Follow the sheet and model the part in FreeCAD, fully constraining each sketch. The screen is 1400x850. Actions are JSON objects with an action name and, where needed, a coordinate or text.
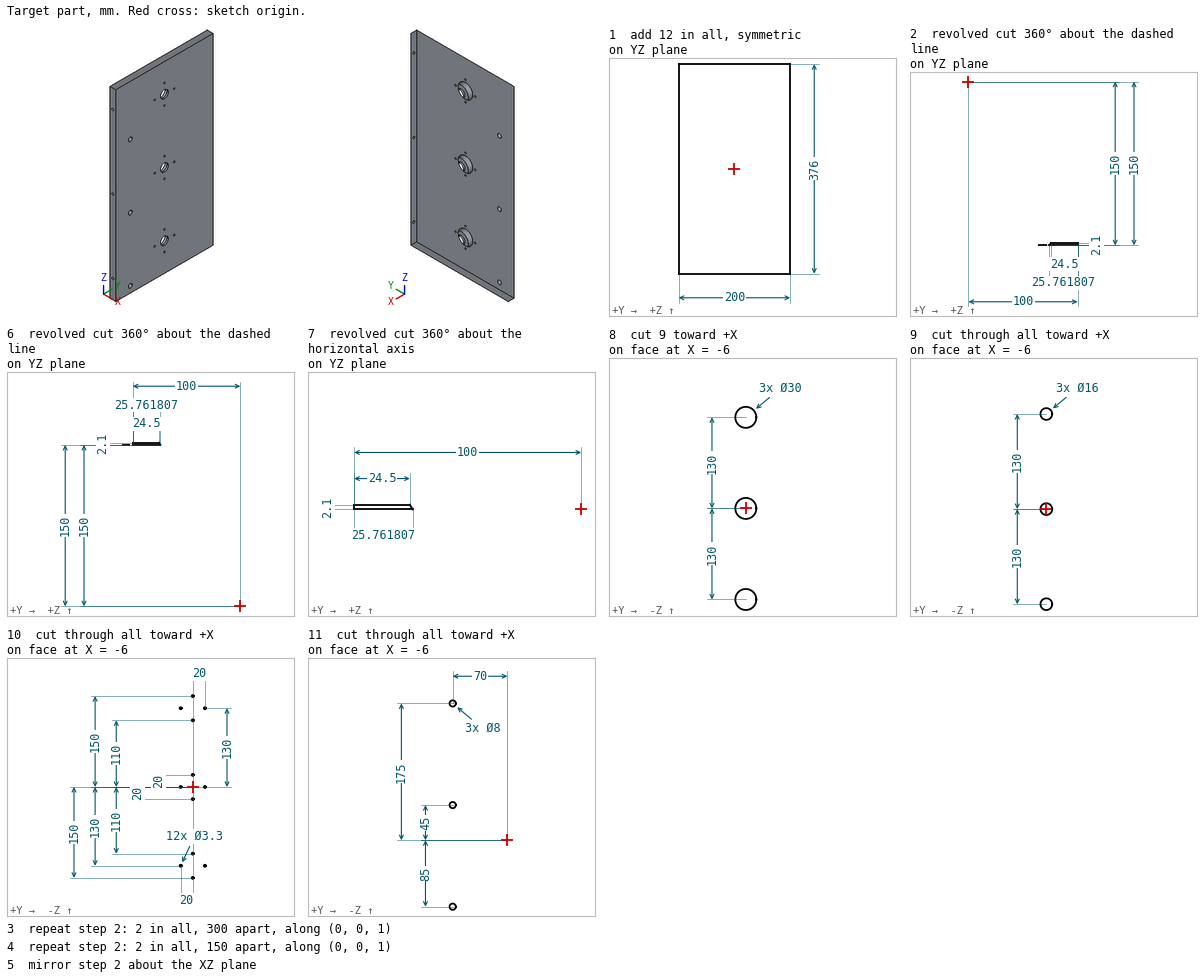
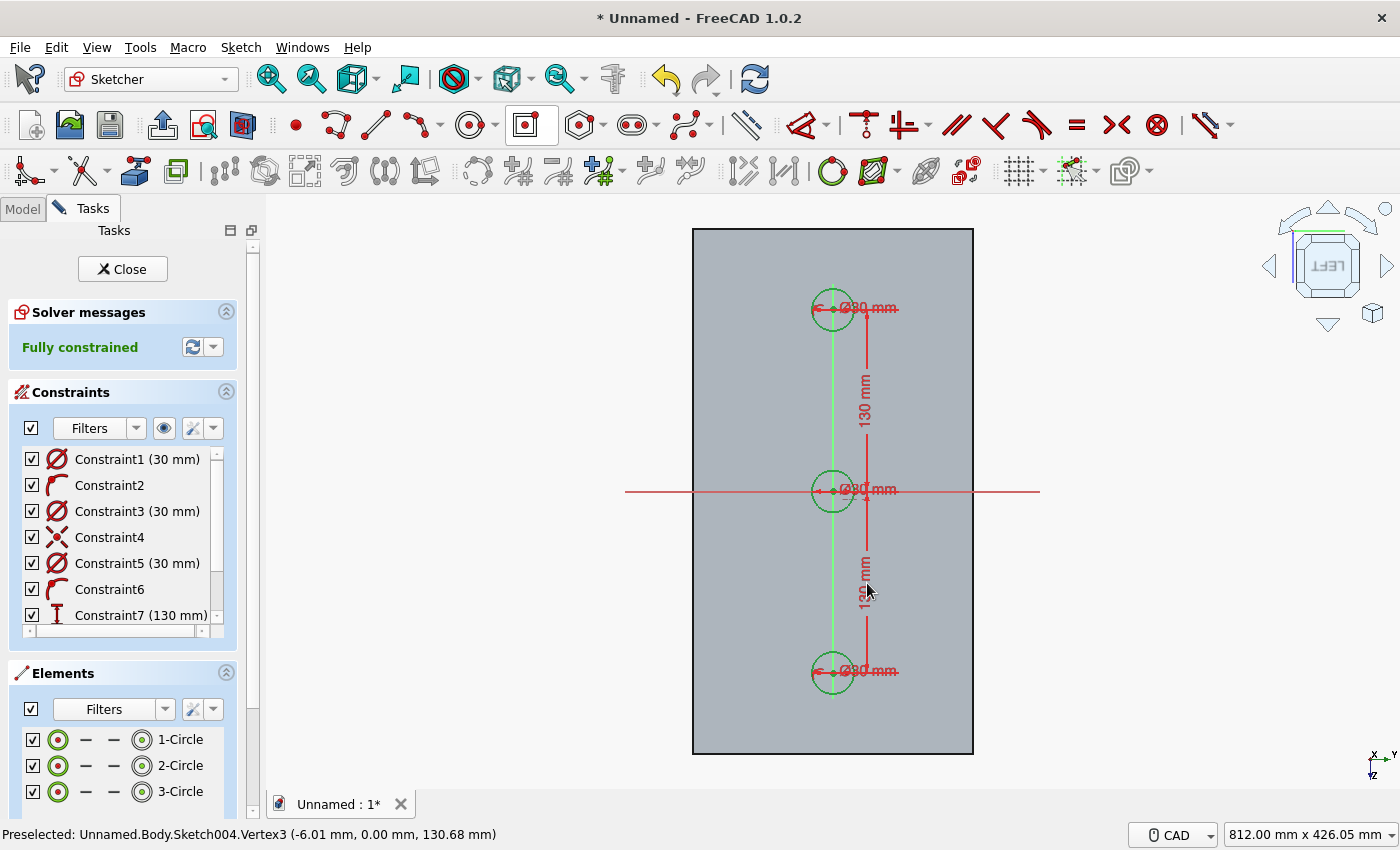
{"action": "left_click", "coordinate": [123, 269]}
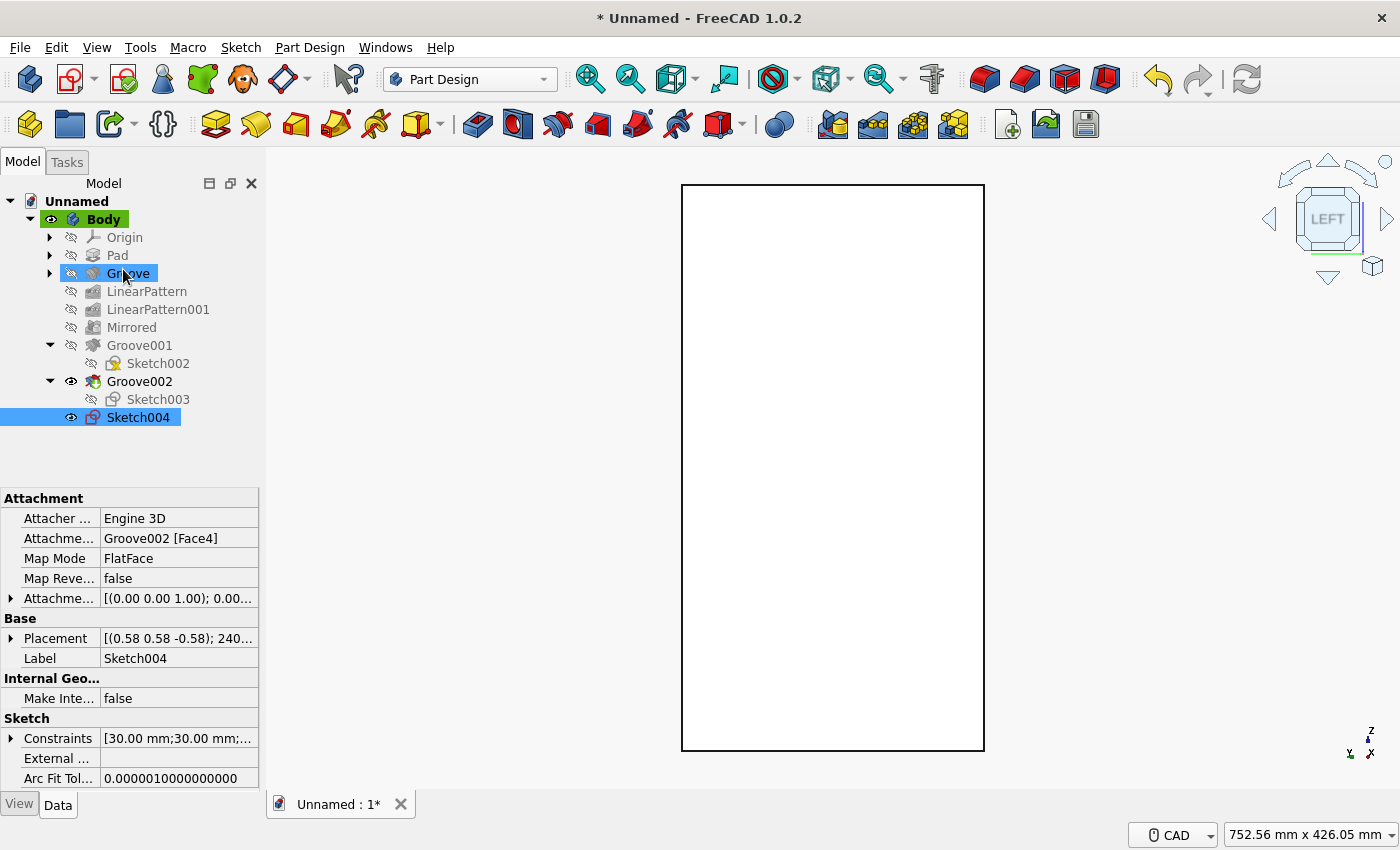
{"action": "left_click", "coordinate": [478, 124]}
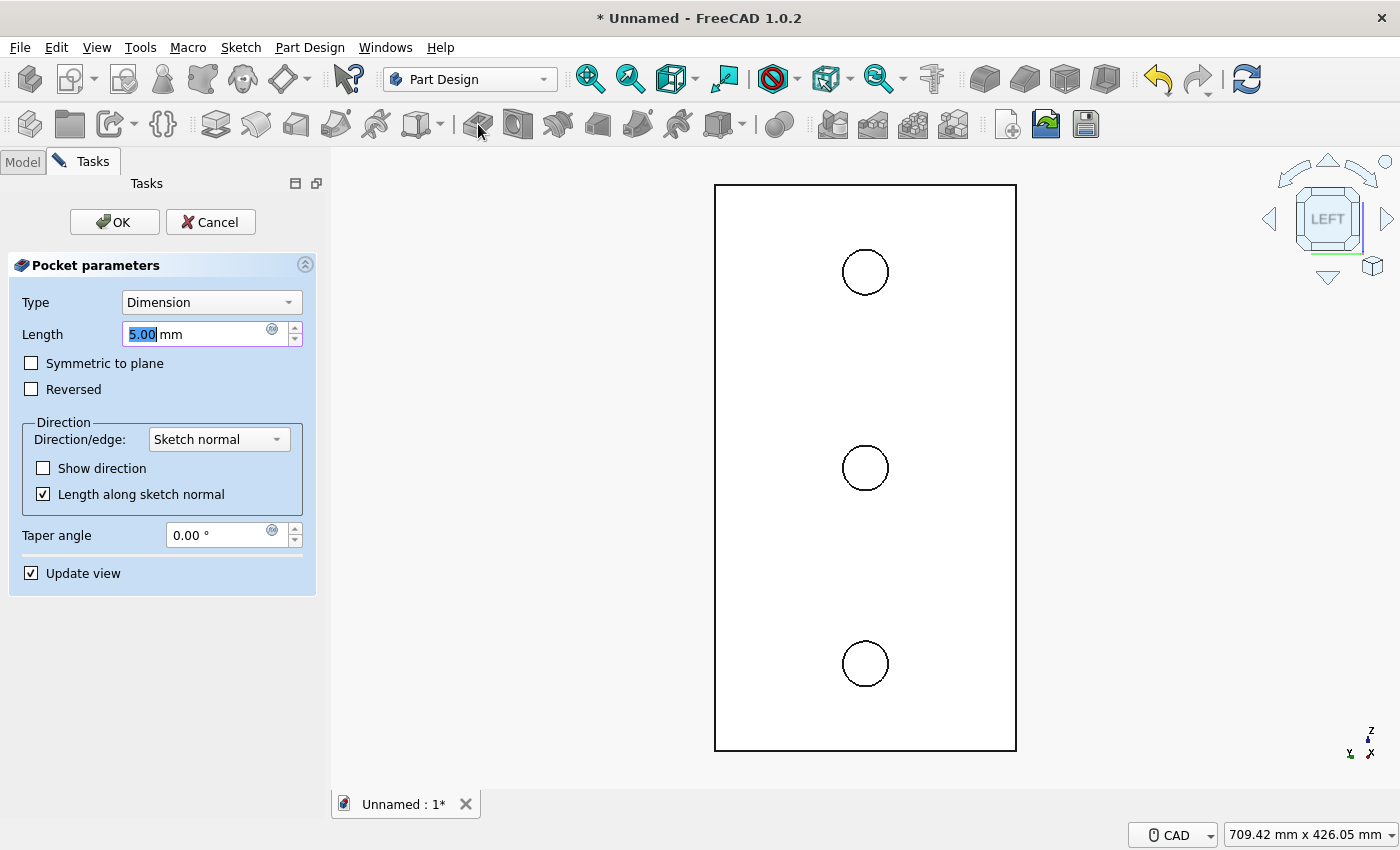
{"action": "type", "text": "9"}
{"action": "key", "text": "Tab"}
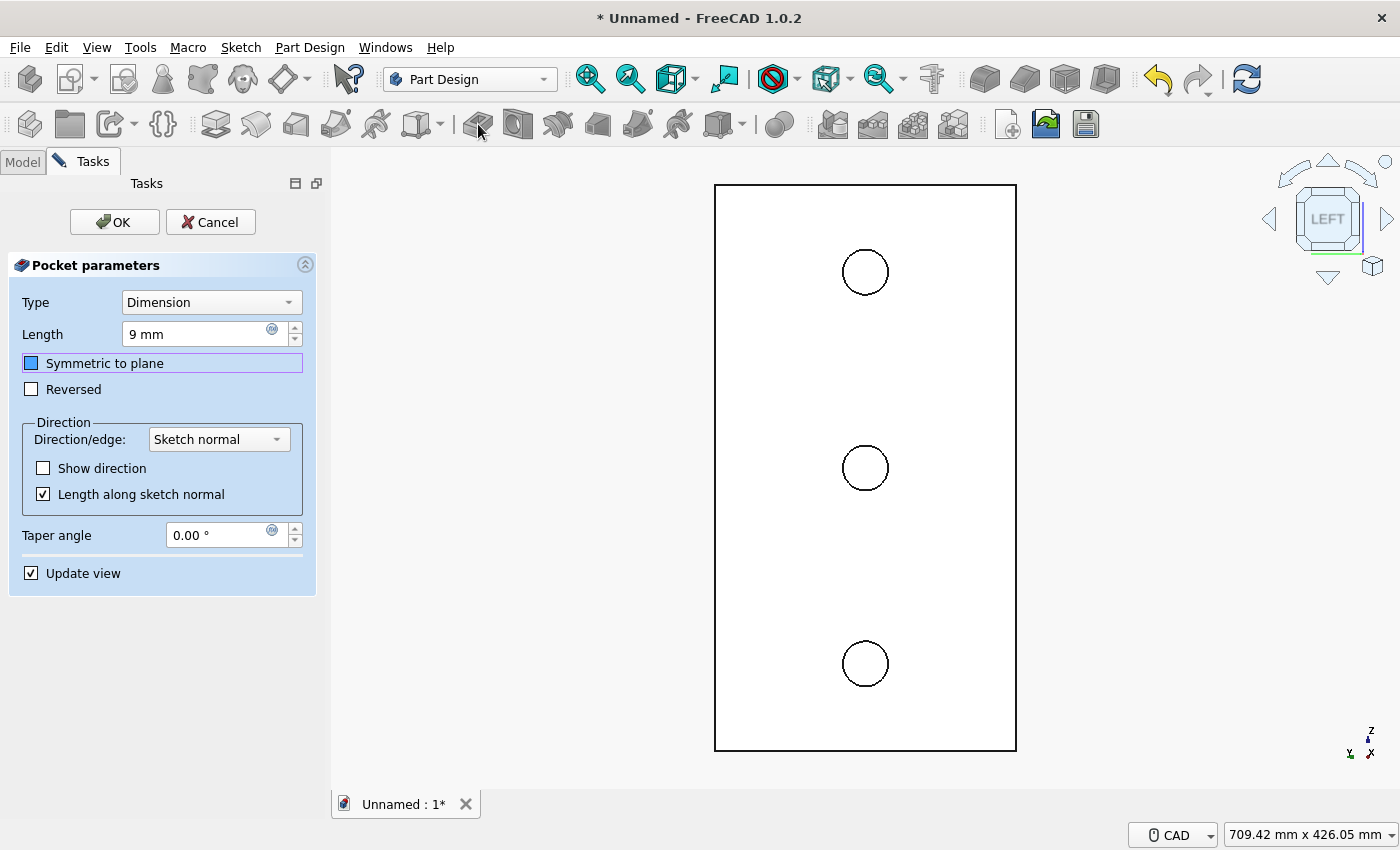
{"action": "left_click", "coordinate": [115, 222]}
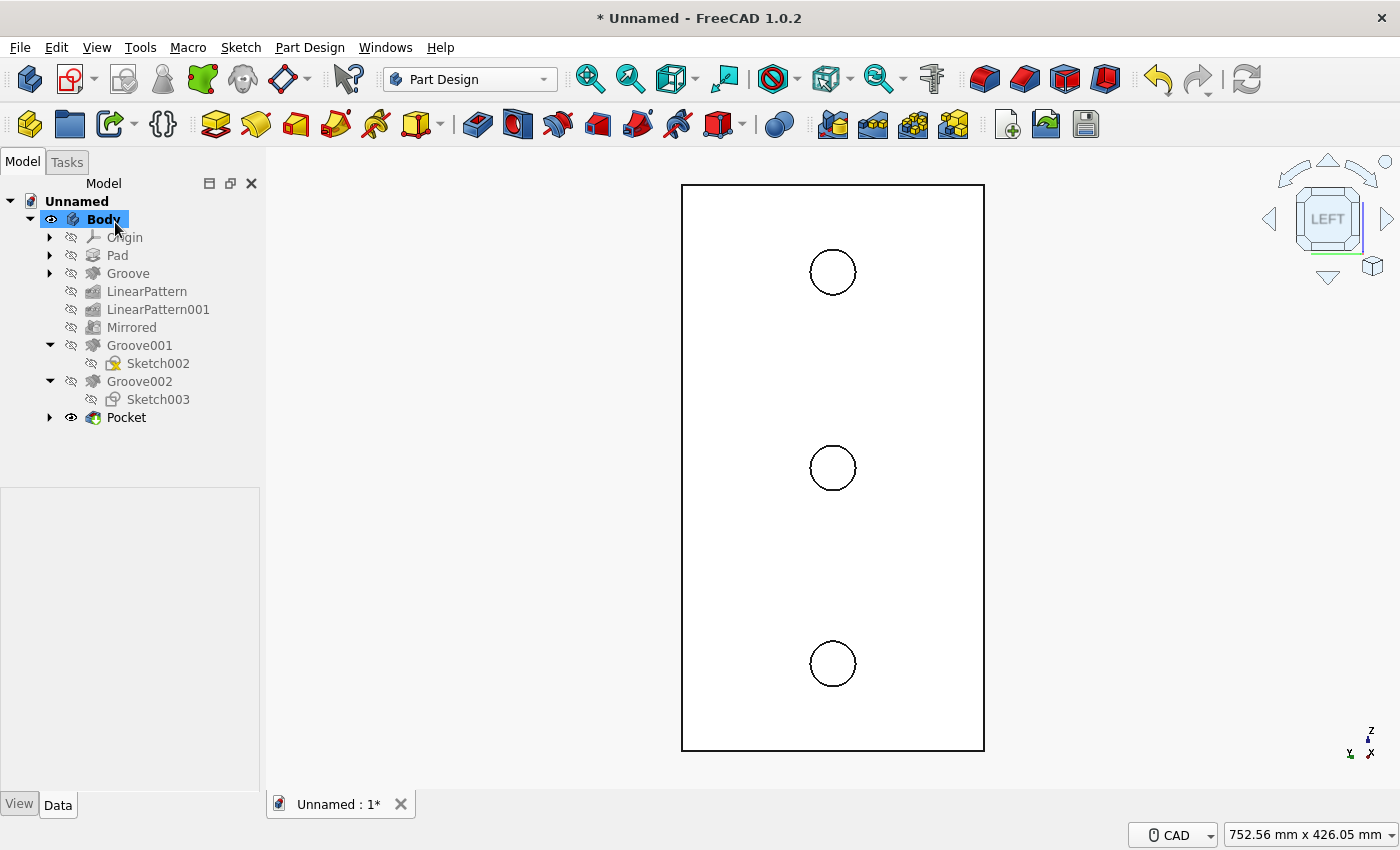
{"action": "left_click", "coordinate": [876, 386]}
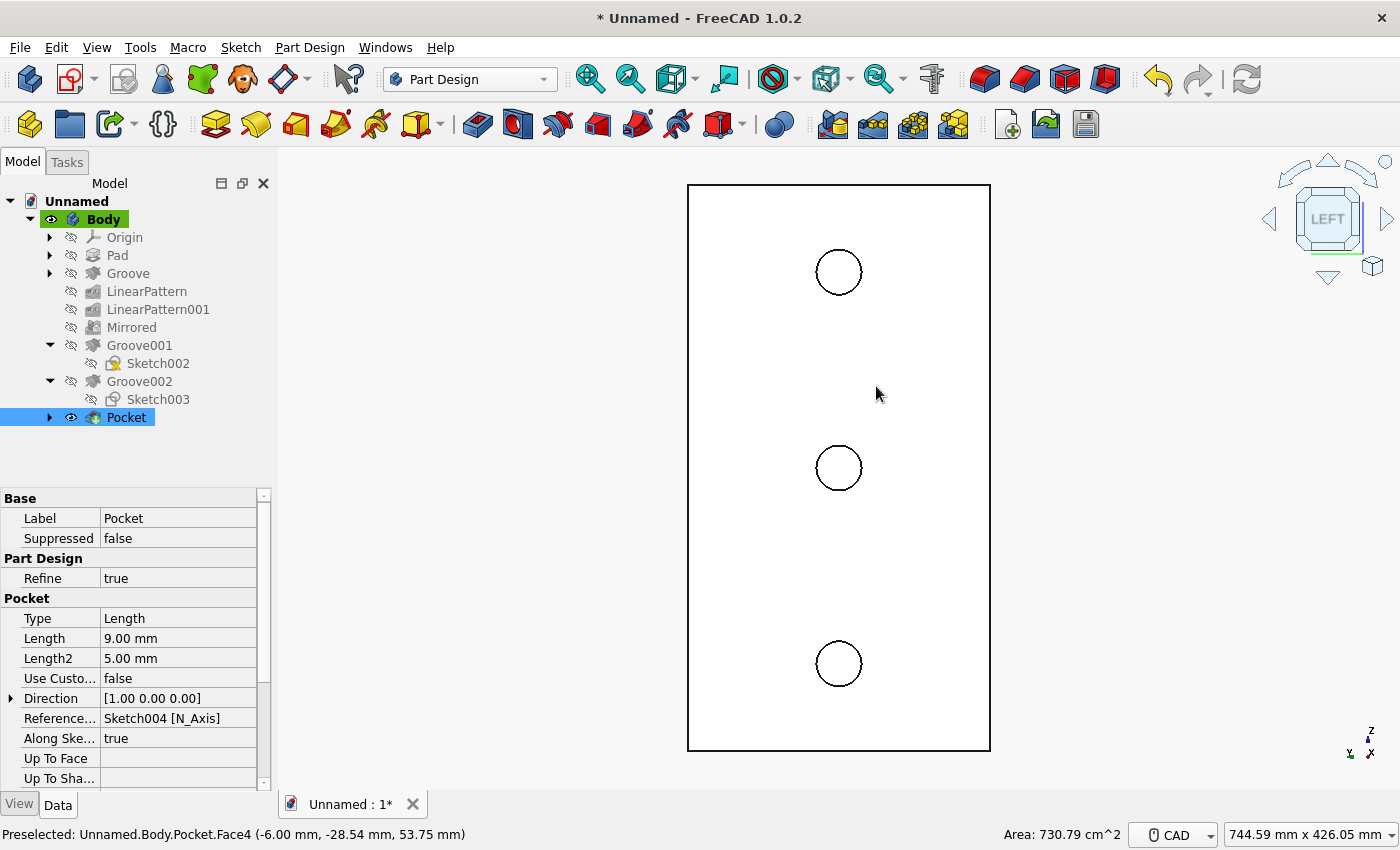
{"action": "left_click", "coordinate": [70, 80]}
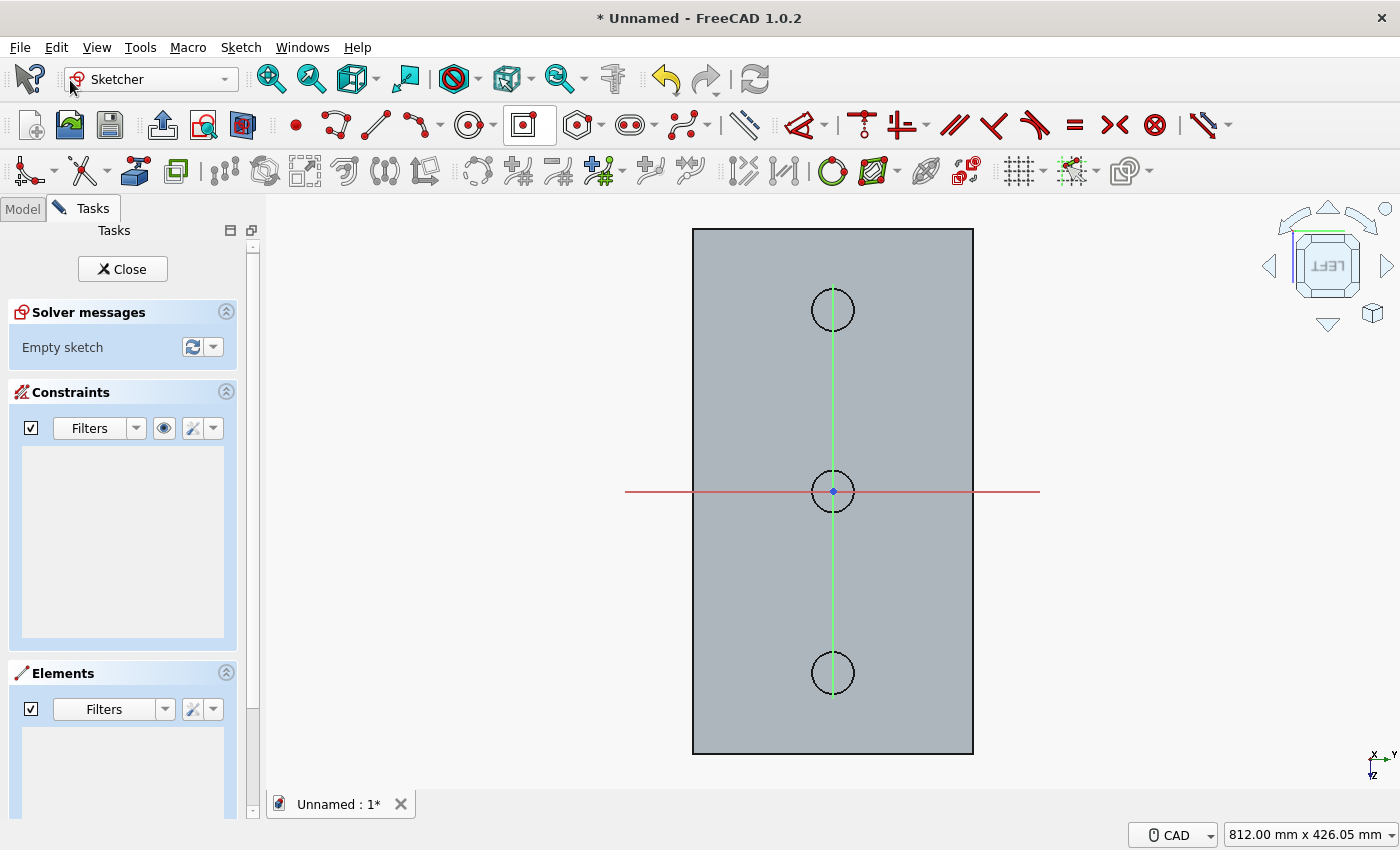
{"action": "left_click", "coordinate": [470, 126]}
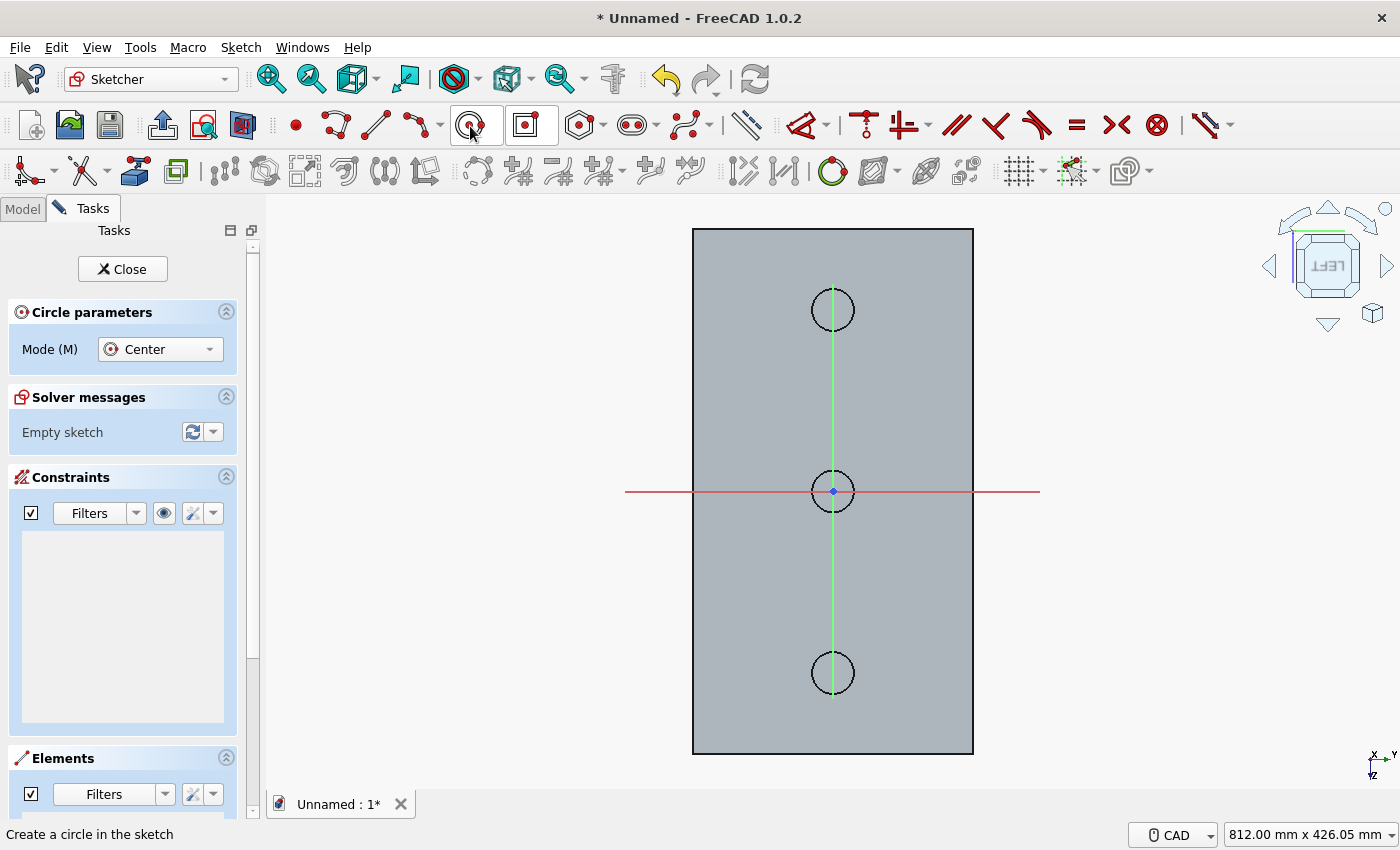
{"action": "scroll", "coordinate": [833, 310], "scroll_direction": "up", "scroll_amount": 4}